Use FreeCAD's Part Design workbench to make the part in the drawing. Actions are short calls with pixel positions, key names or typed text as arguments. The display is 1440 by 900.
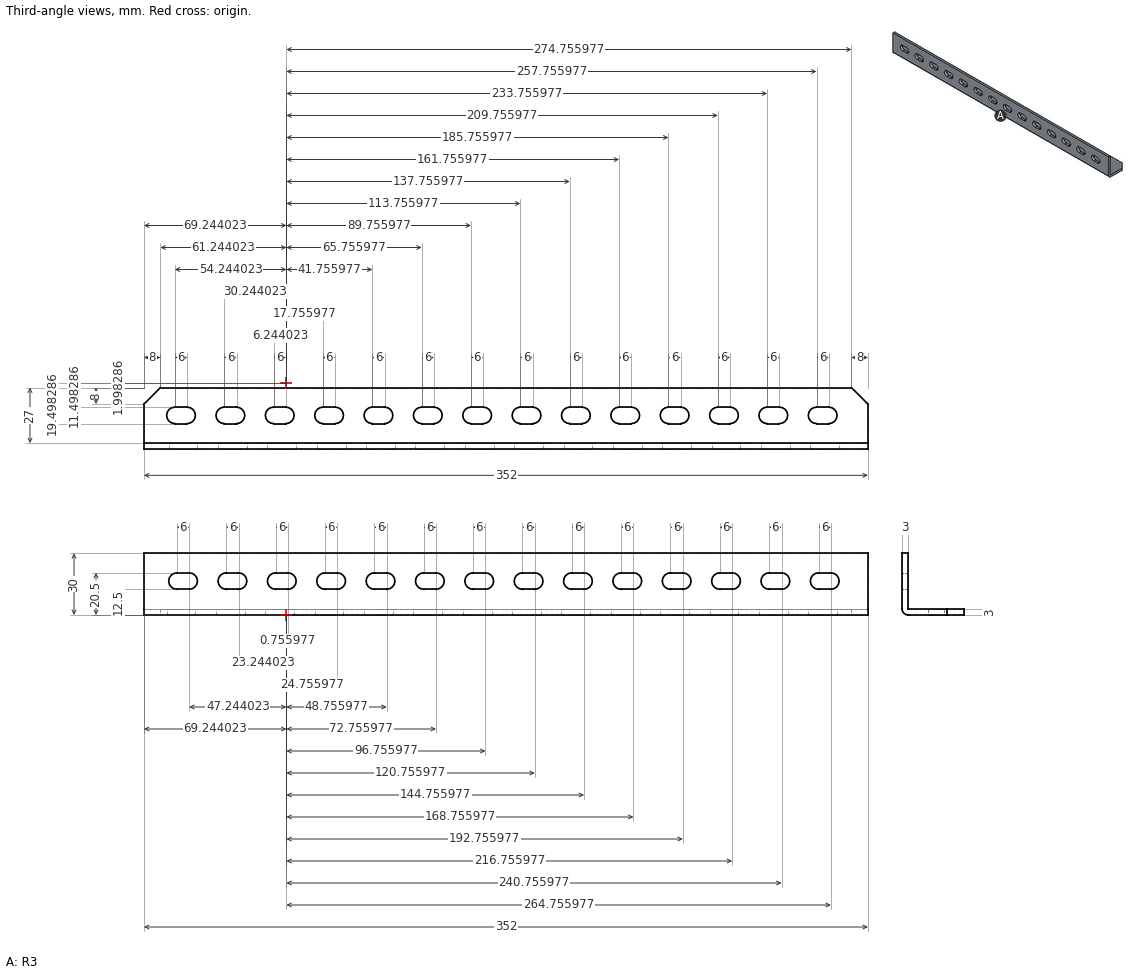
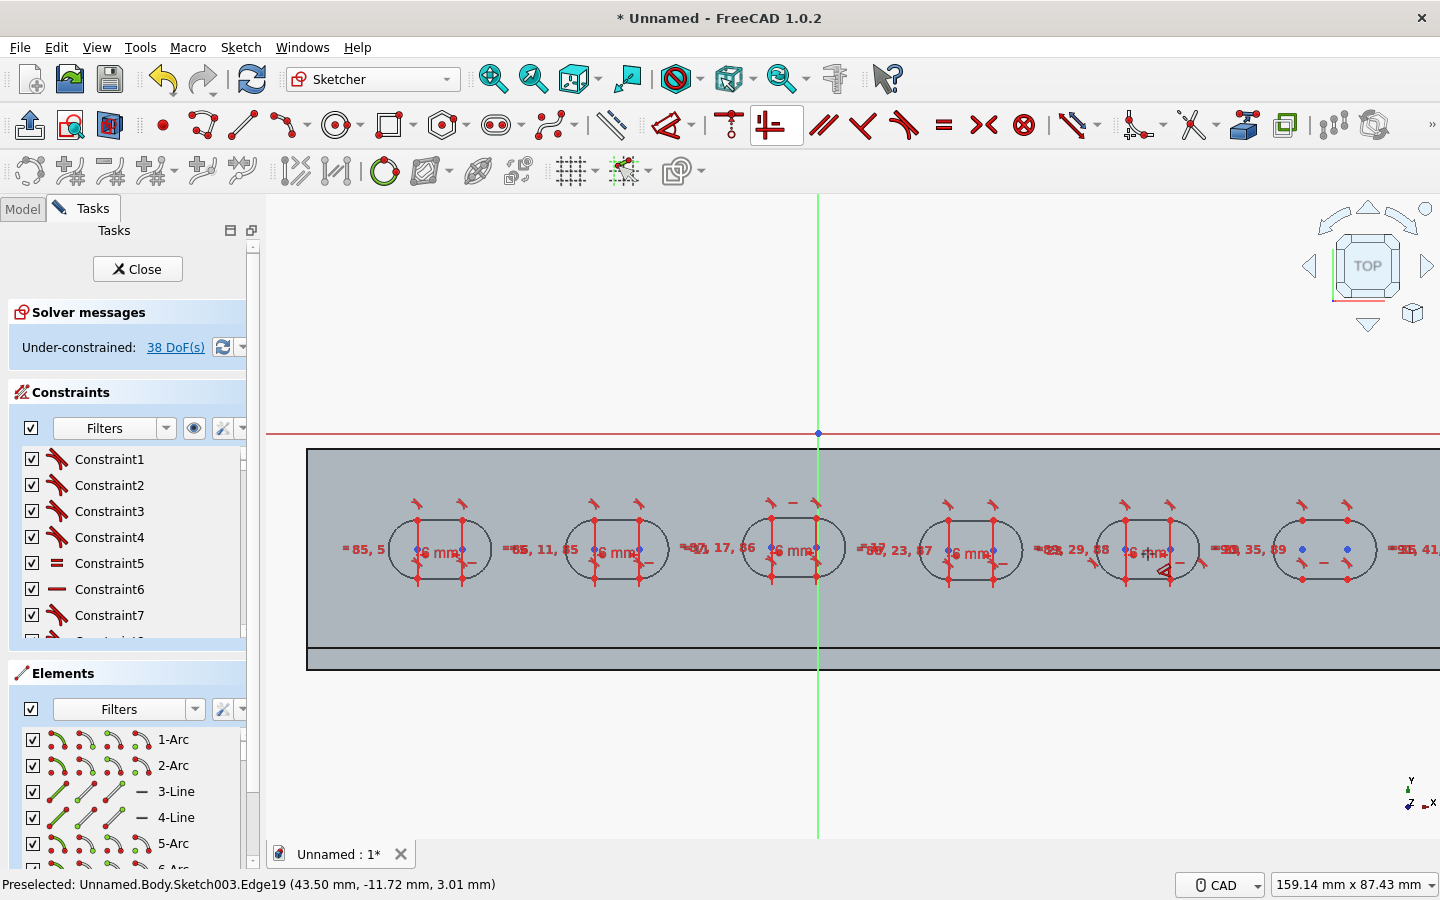
scroll(437, 521, down, 6)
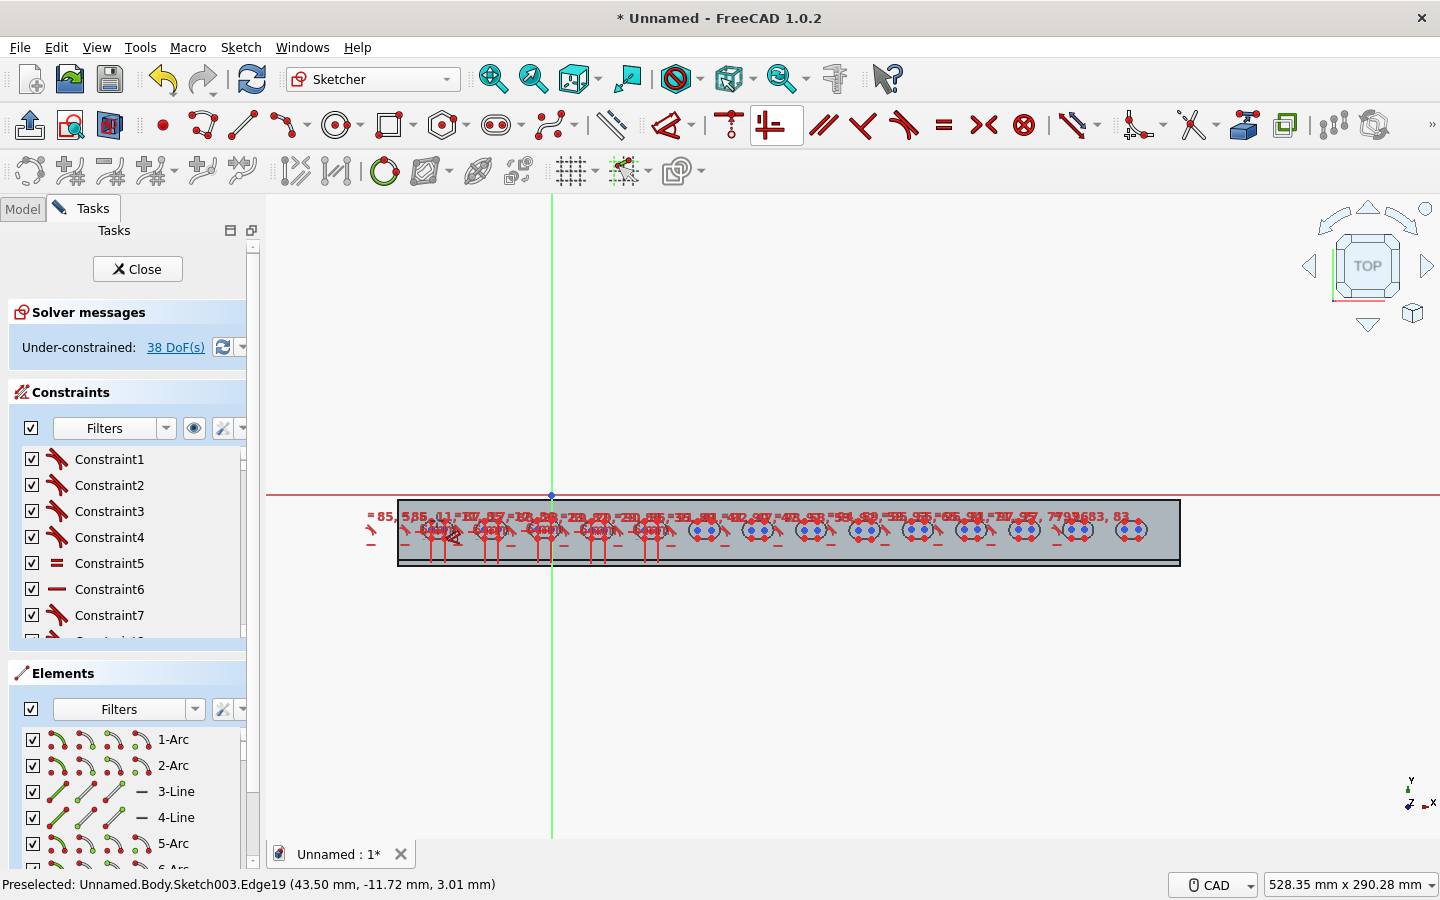
scroll(702, 521, up, 7)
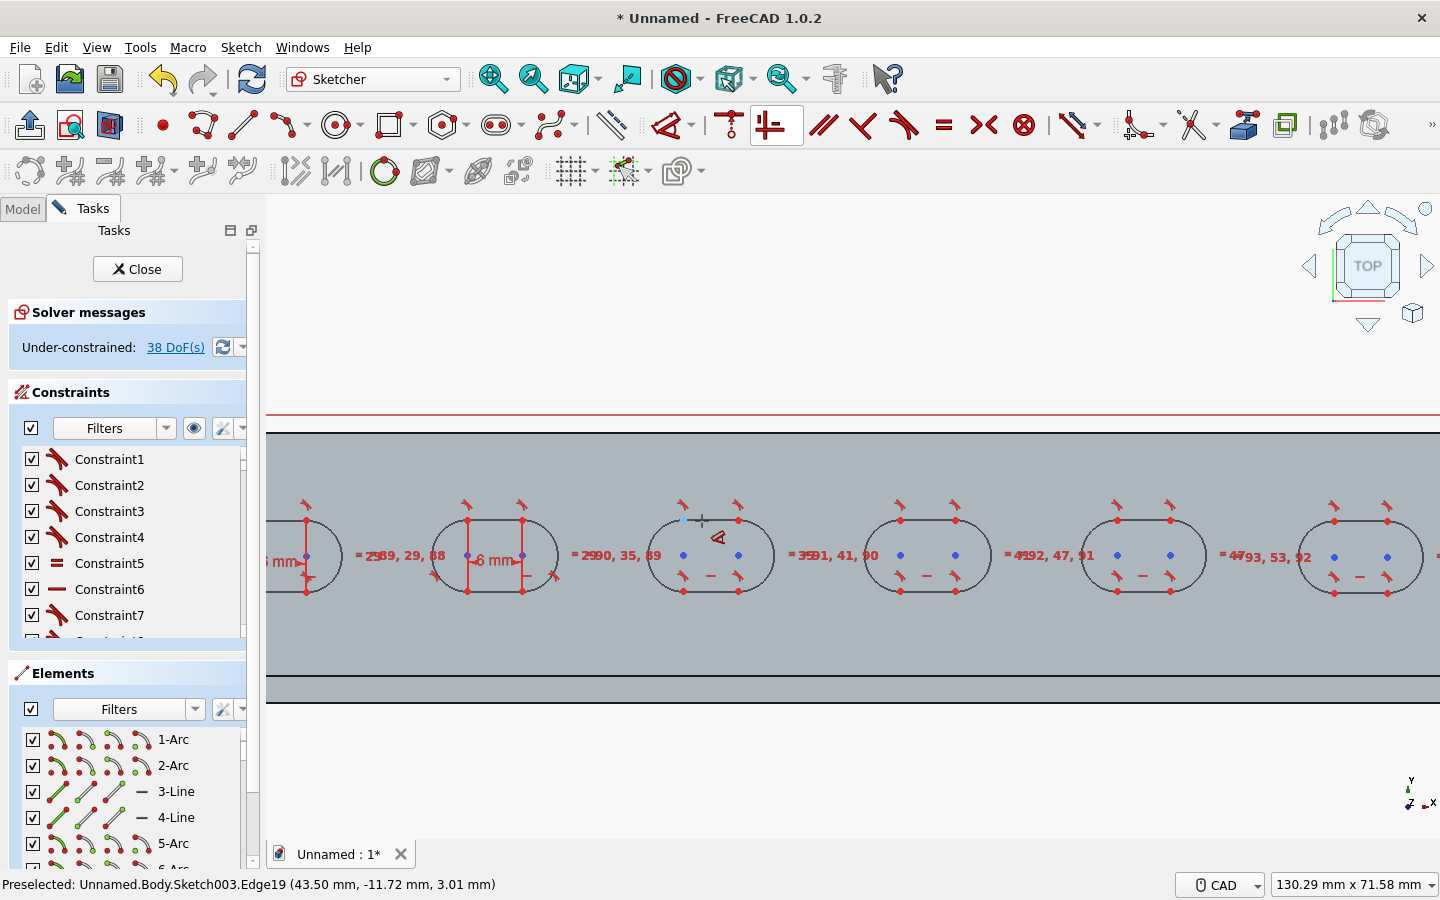
click(700, 520)
click(711, 554)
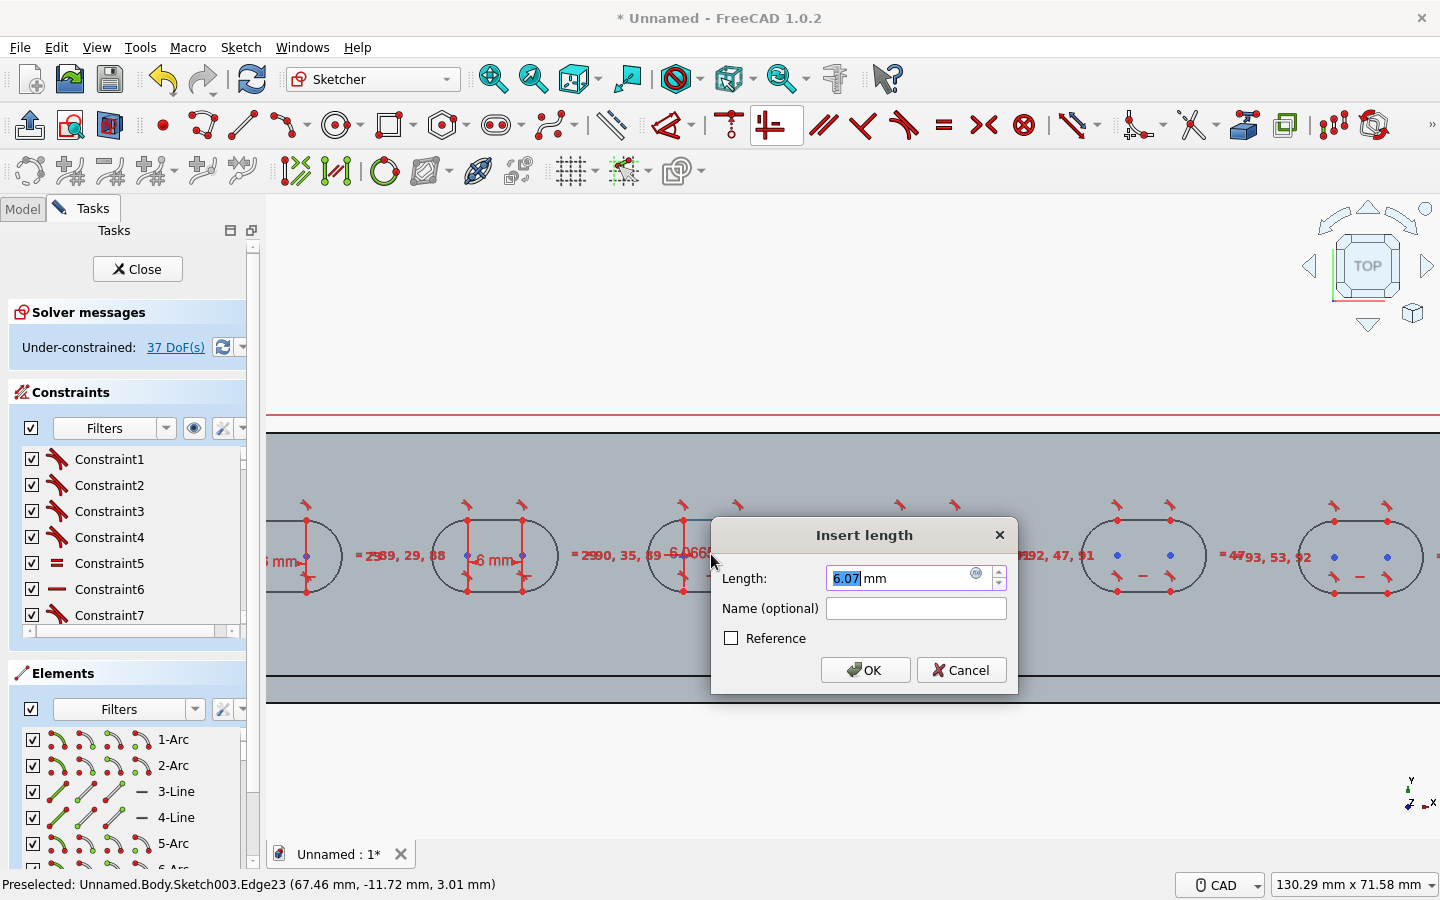
text(6)
key(Return)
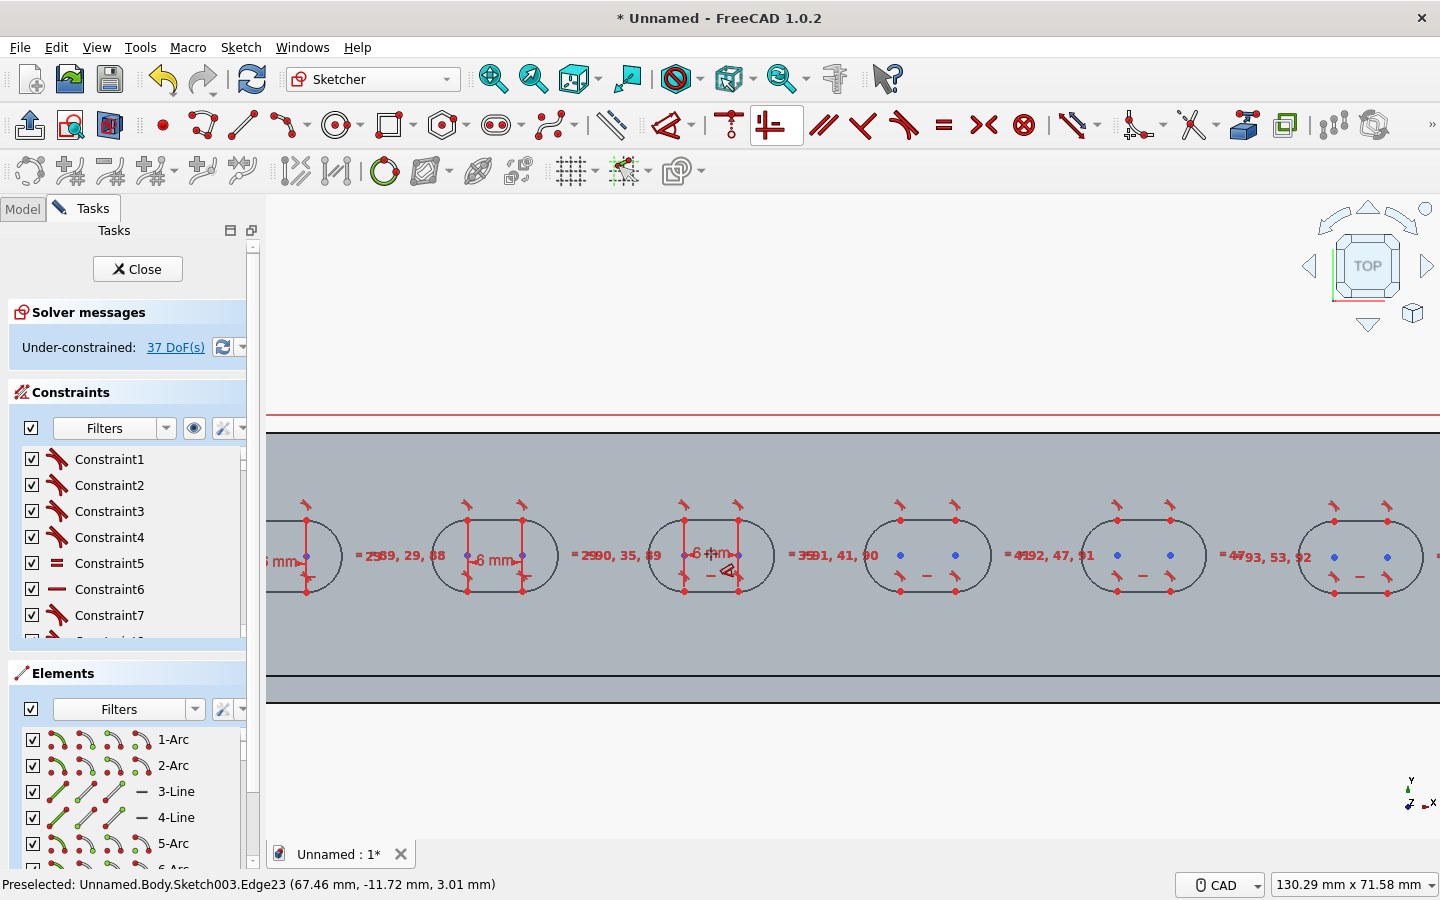
click(917, 520)
click(928, 554)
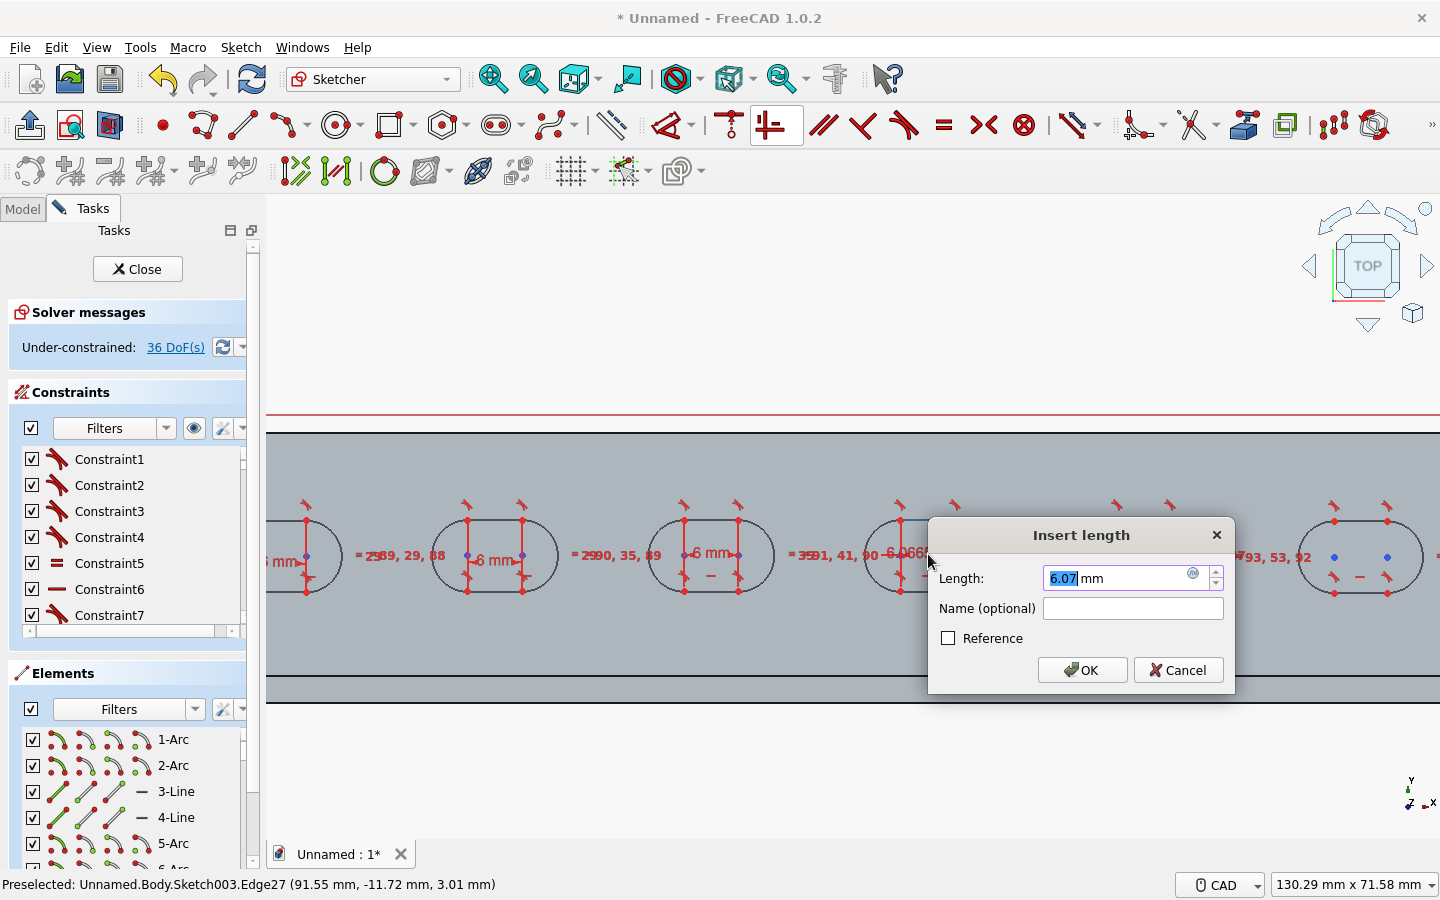
text(6)
key(Return)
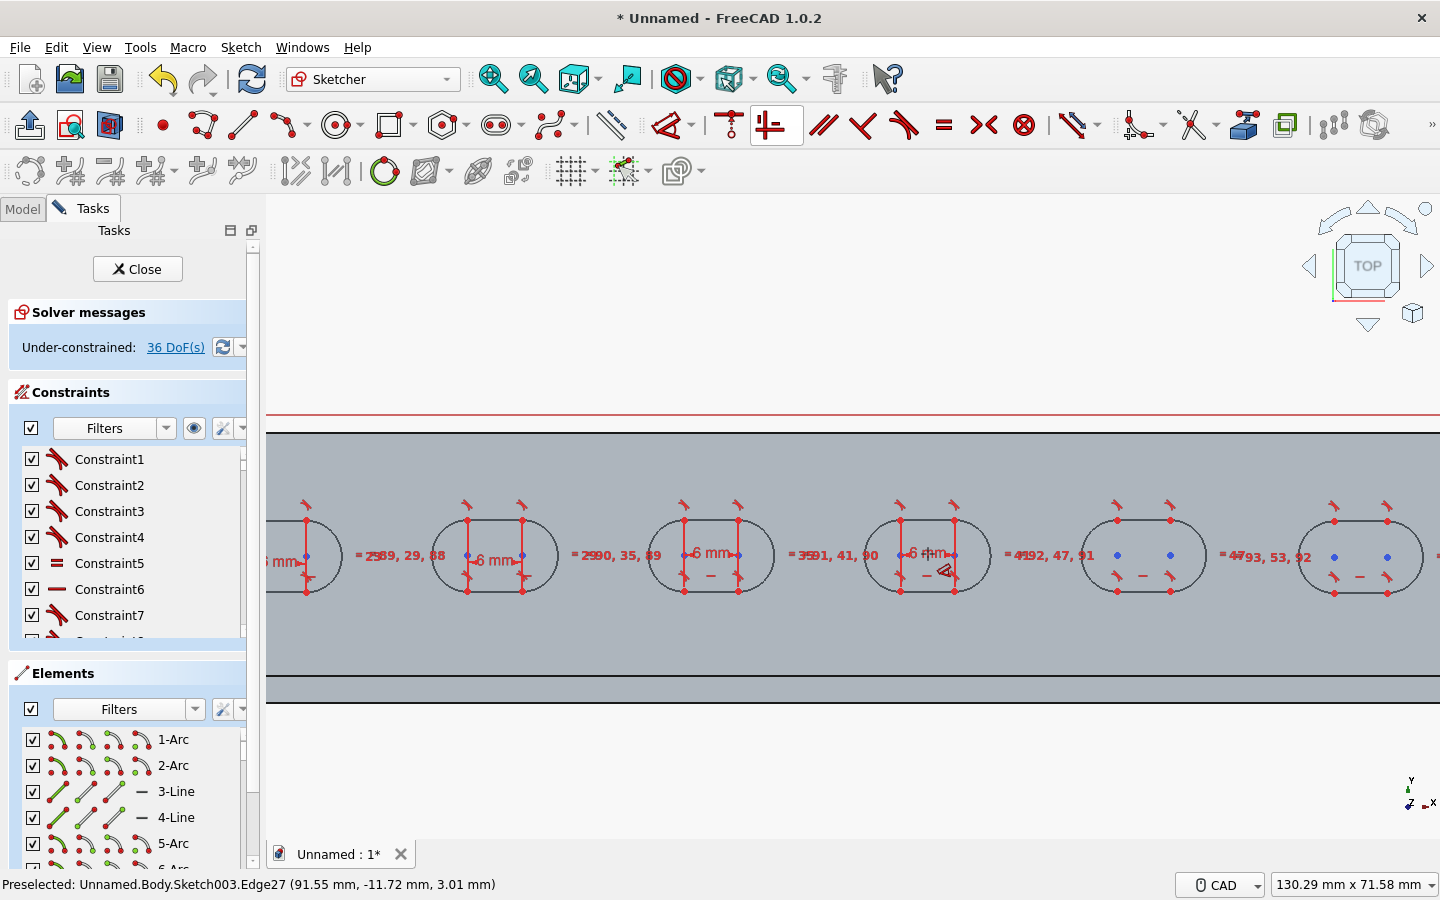
click(1133, 520)
click(1144, 554)